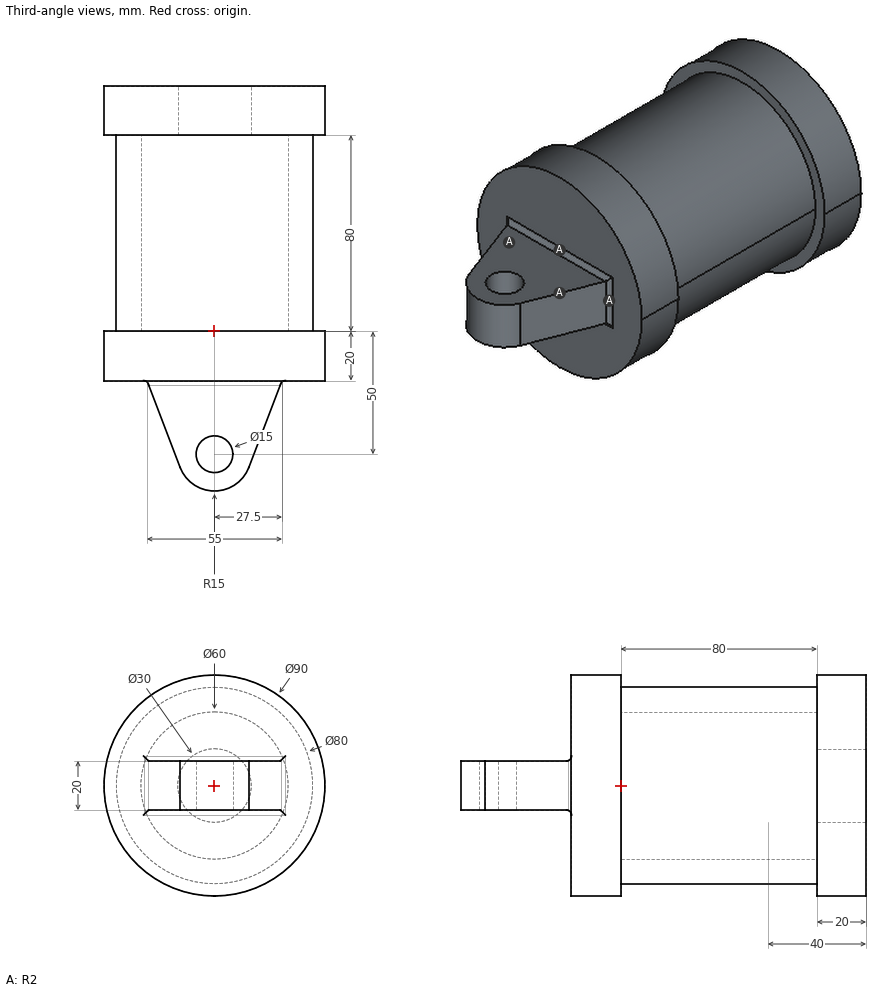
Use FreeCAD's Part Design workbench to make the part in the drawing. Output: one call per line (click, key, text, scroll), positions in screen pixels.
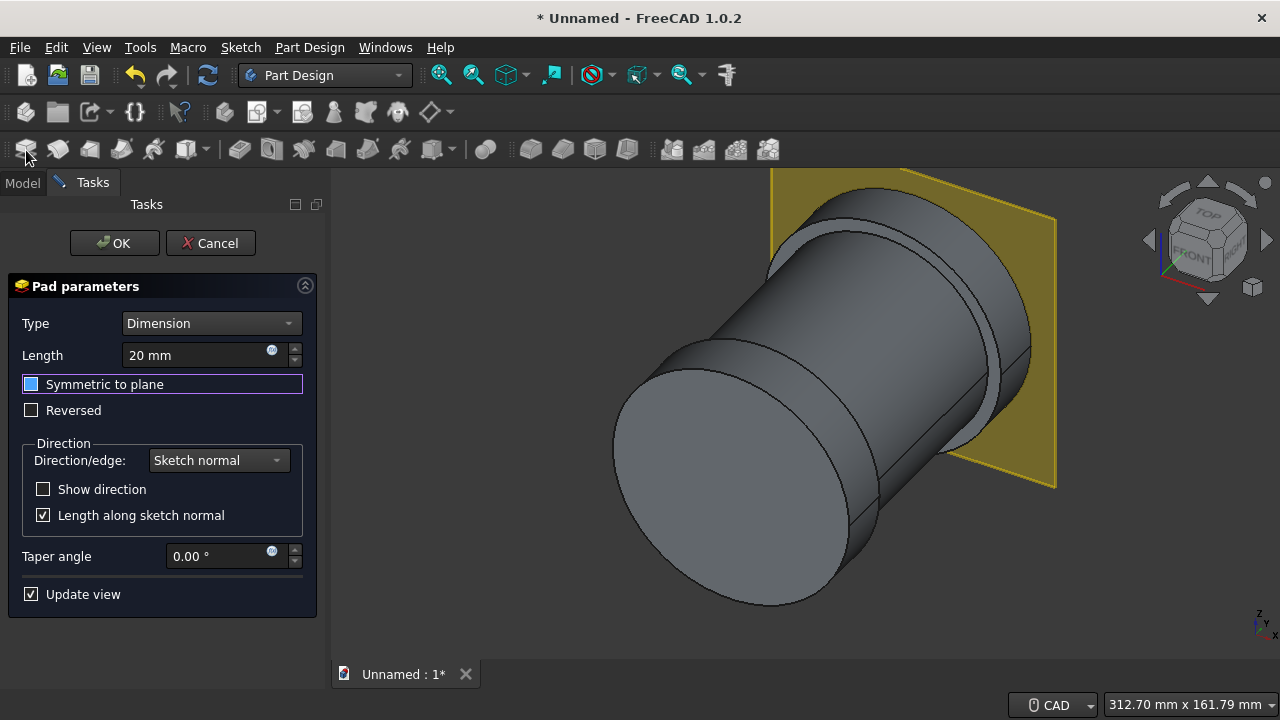
click(115, 243)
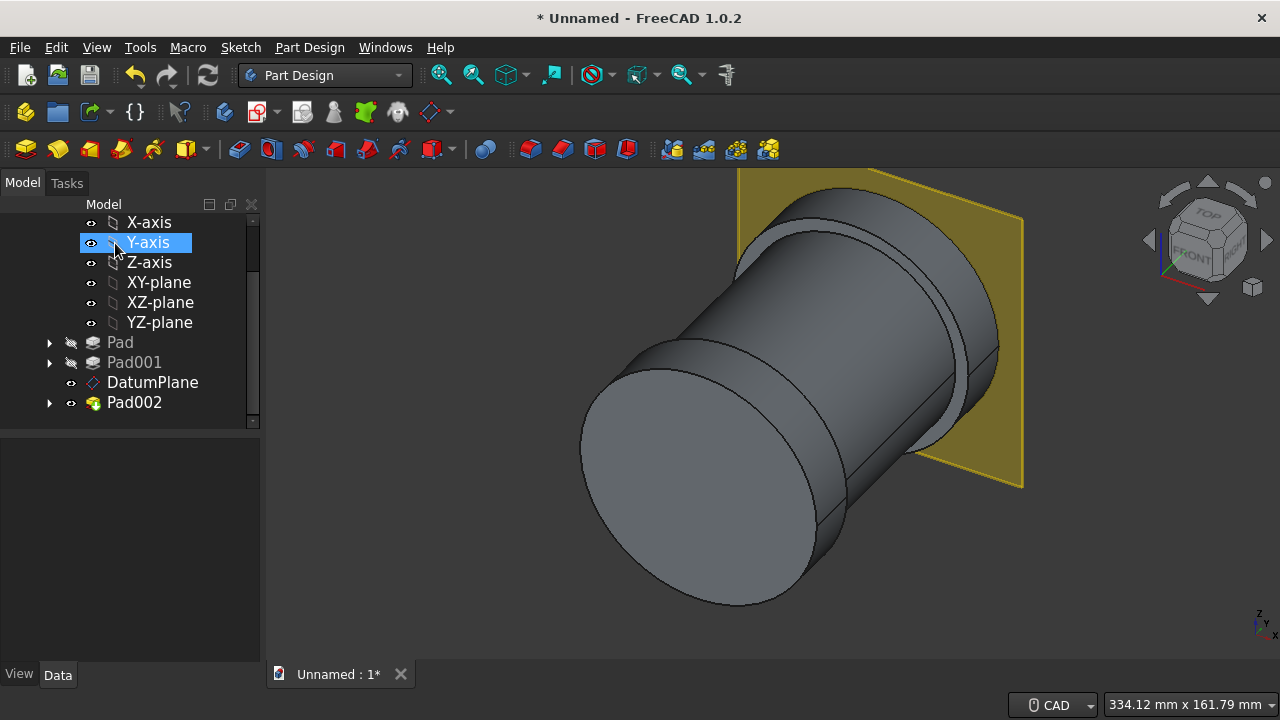
click(116, 383)
key(space)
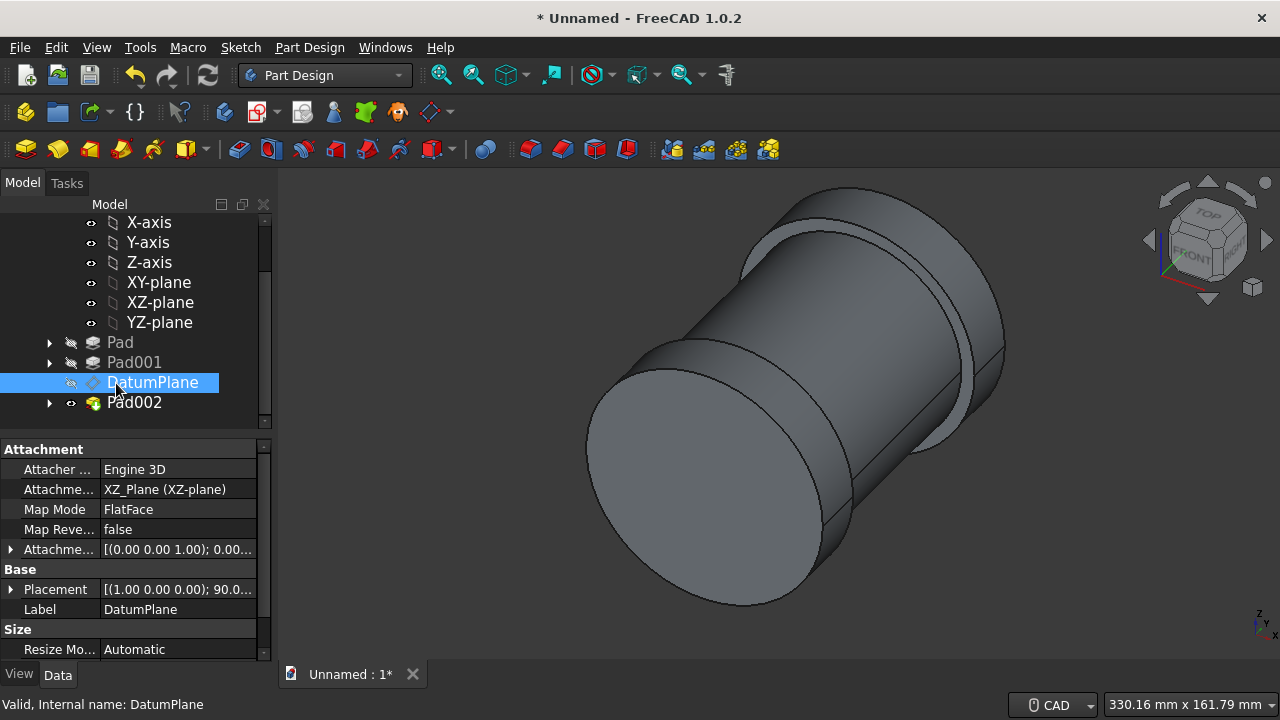
key(v)
key(f)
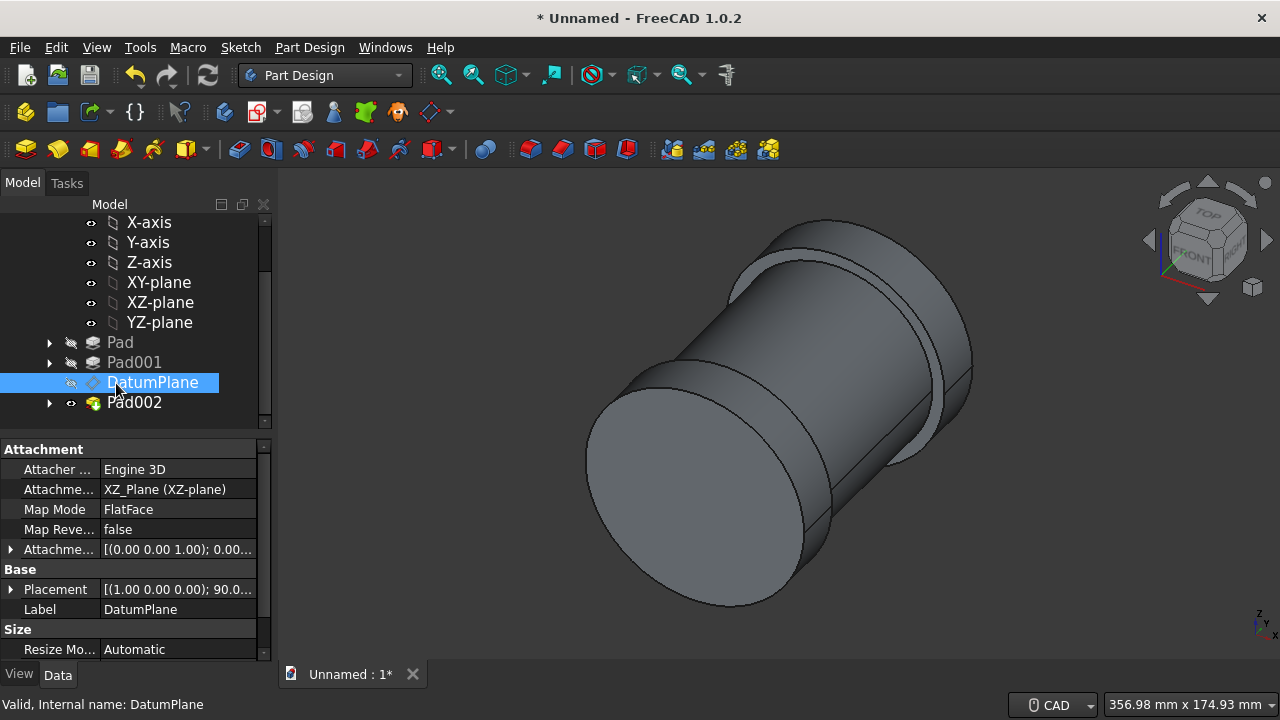
scroll(160, 318, down, 3)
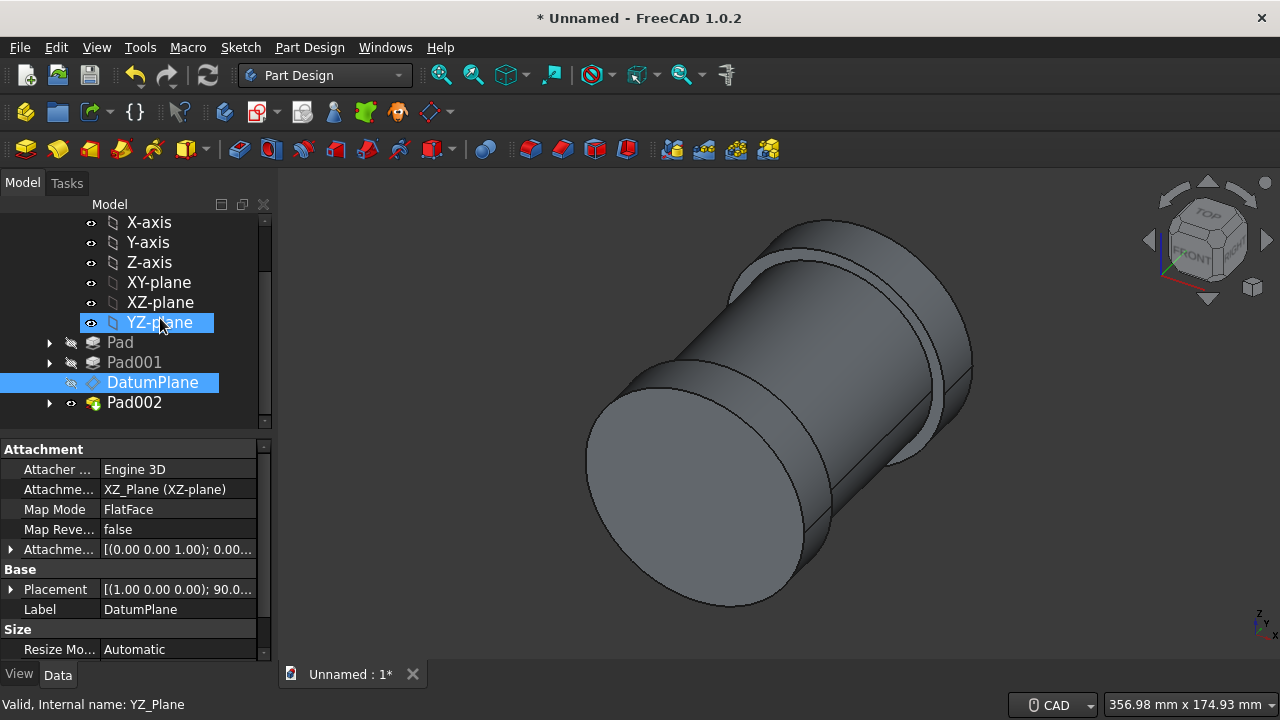
scroll(160, 318, up, 15)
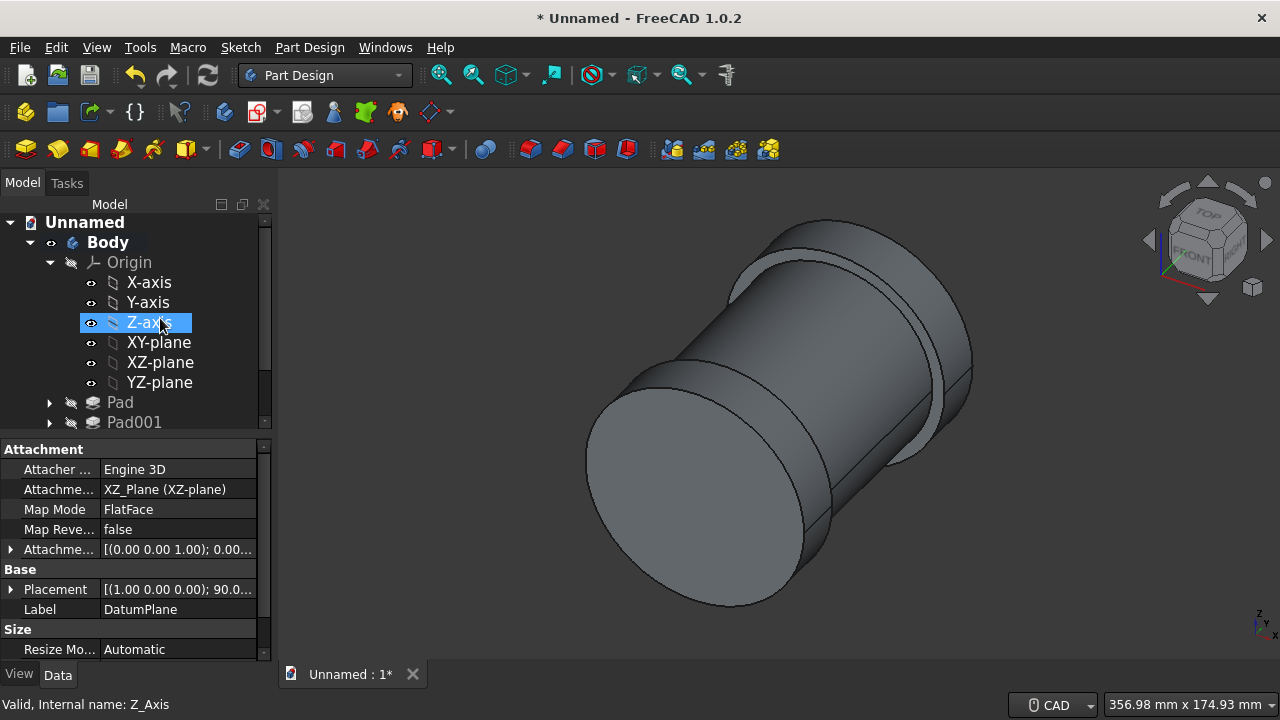
click(136, 363)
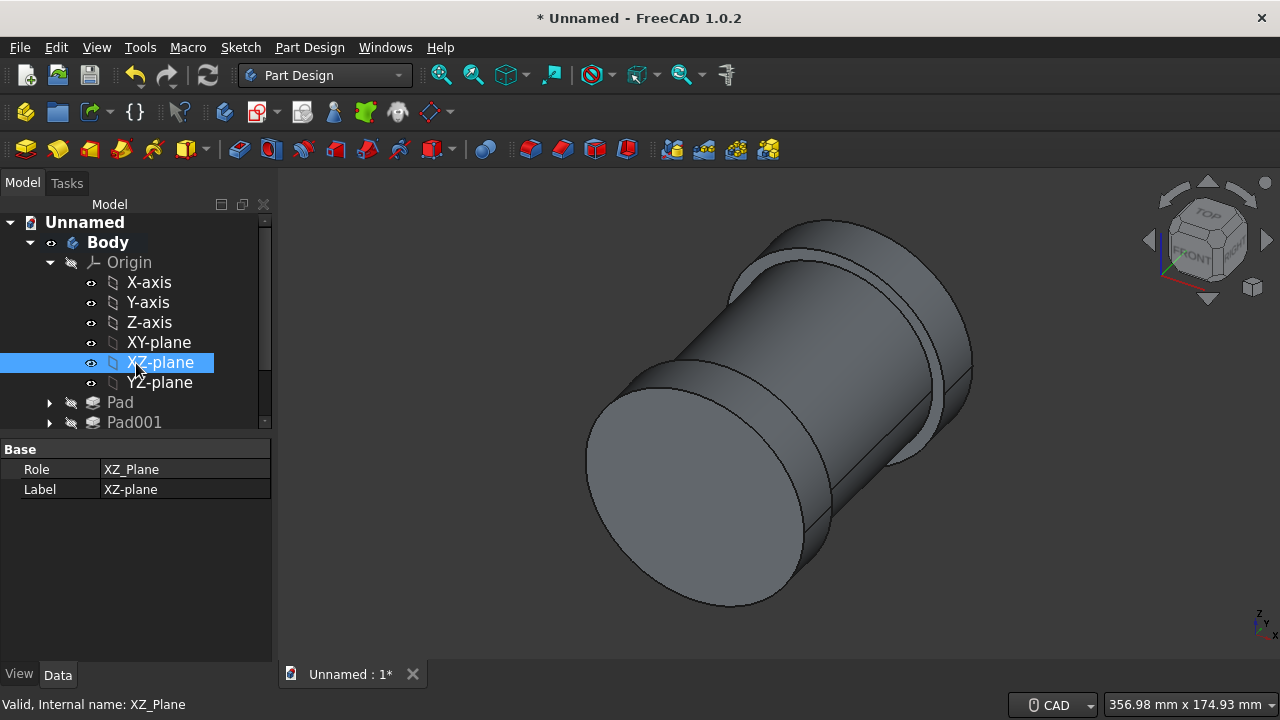
click(430, 112)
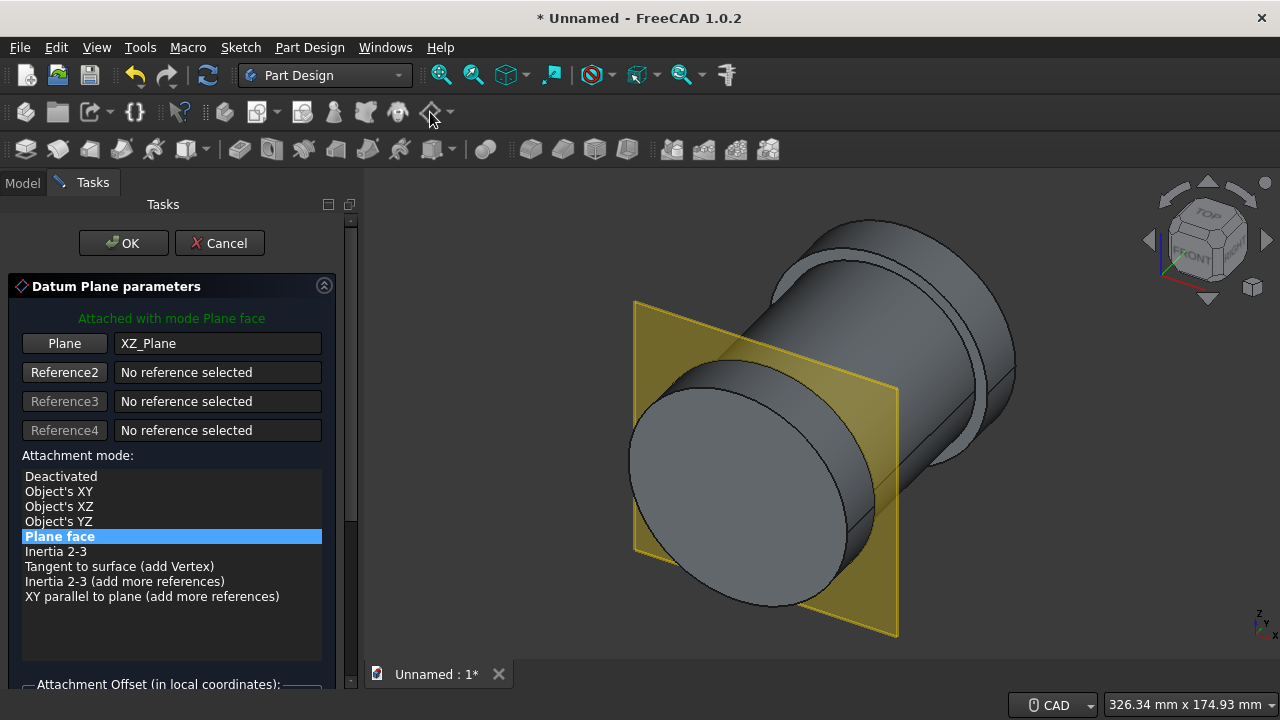
scroll(351, 451, down, 3)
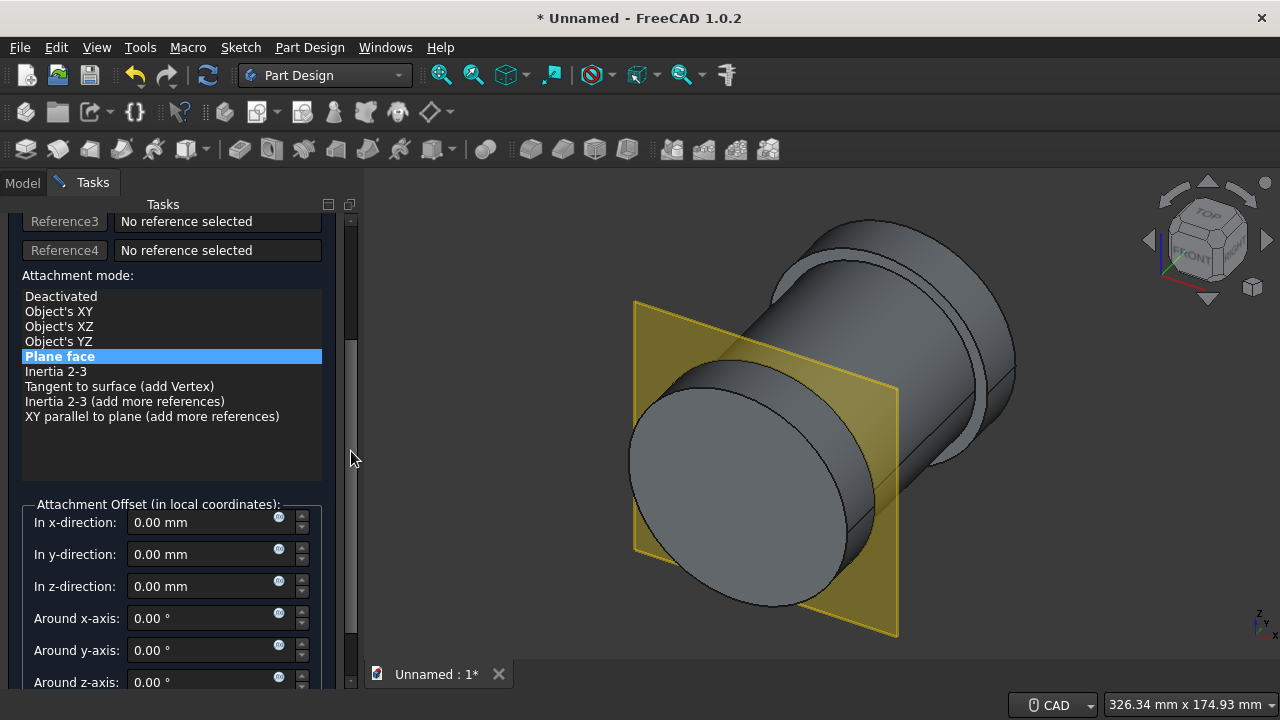
triple_click(210, 586)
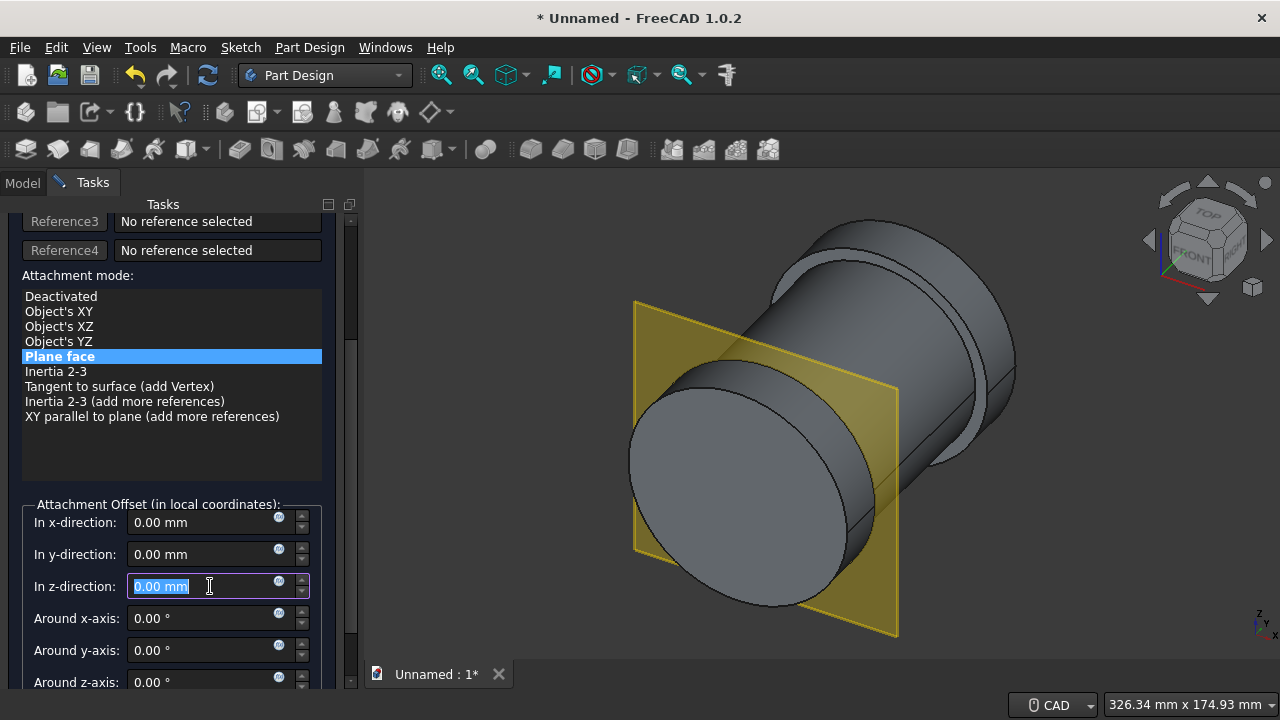
text(-80)
key(Tab)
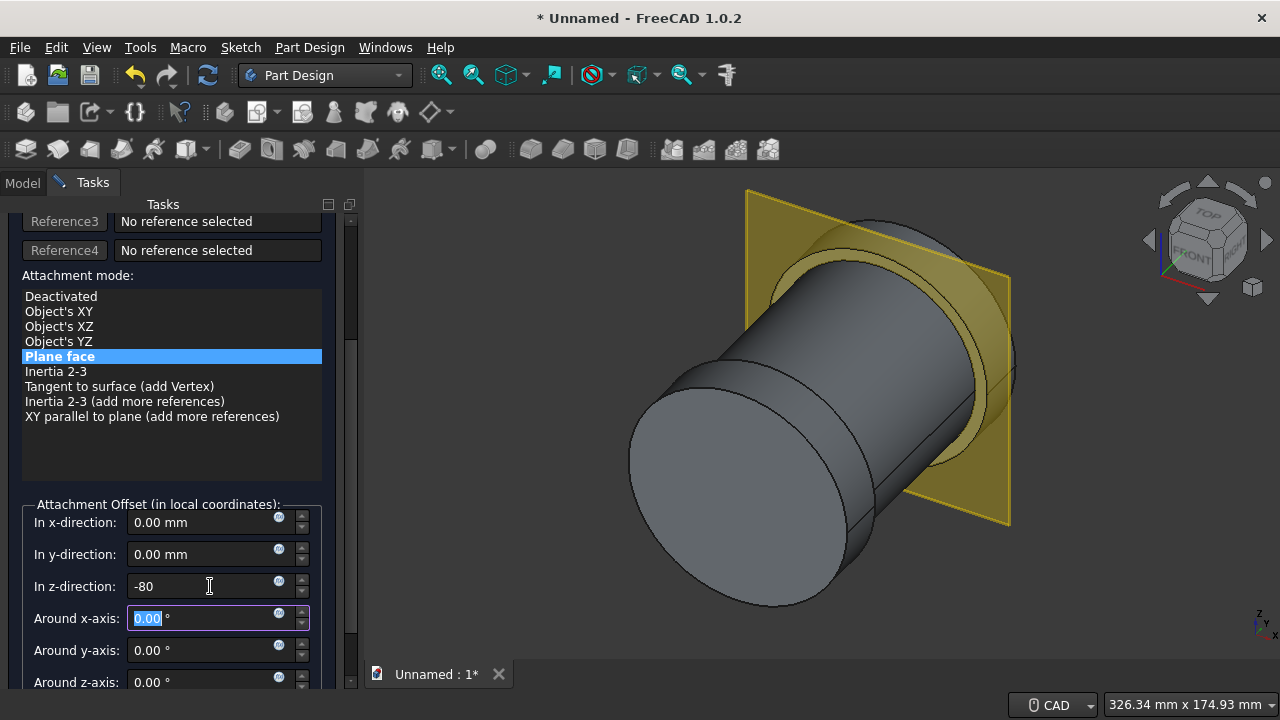
scroll(351, 451, up, 4)